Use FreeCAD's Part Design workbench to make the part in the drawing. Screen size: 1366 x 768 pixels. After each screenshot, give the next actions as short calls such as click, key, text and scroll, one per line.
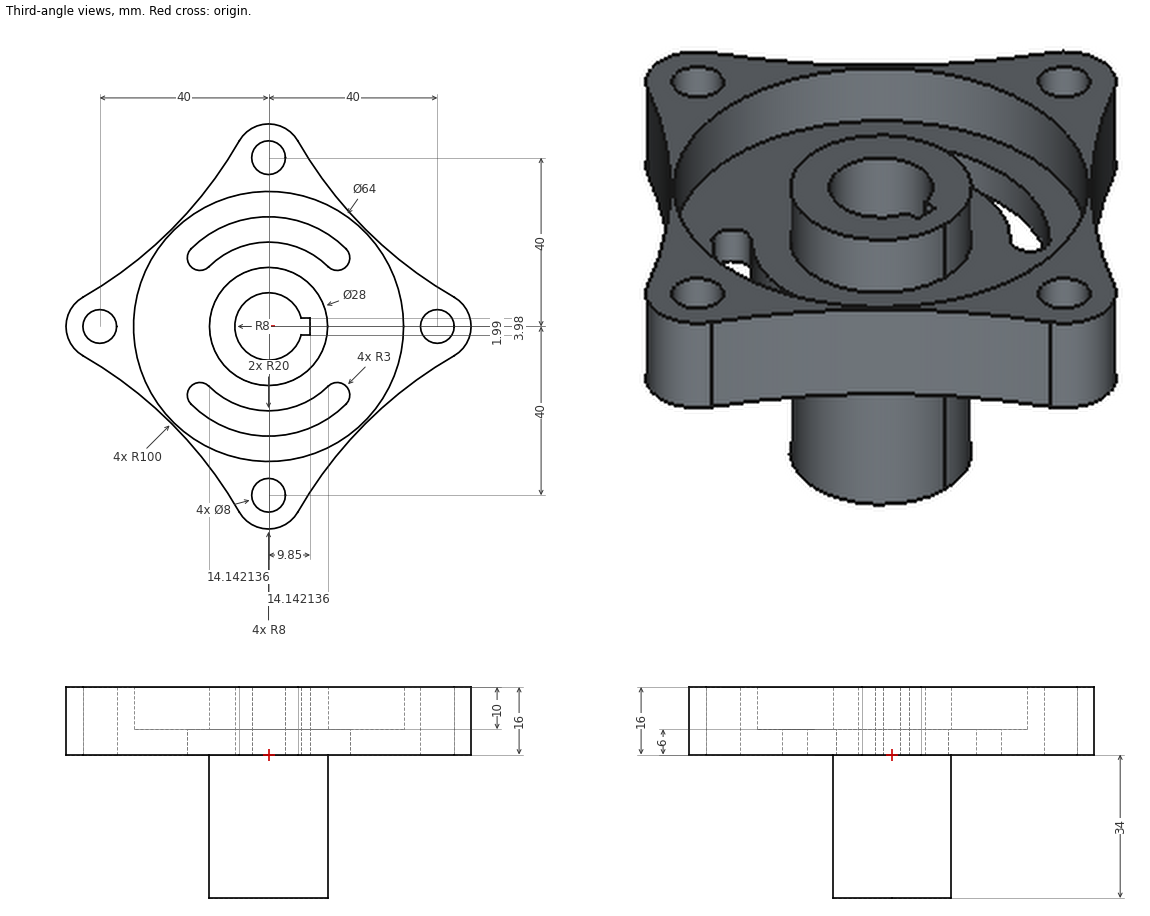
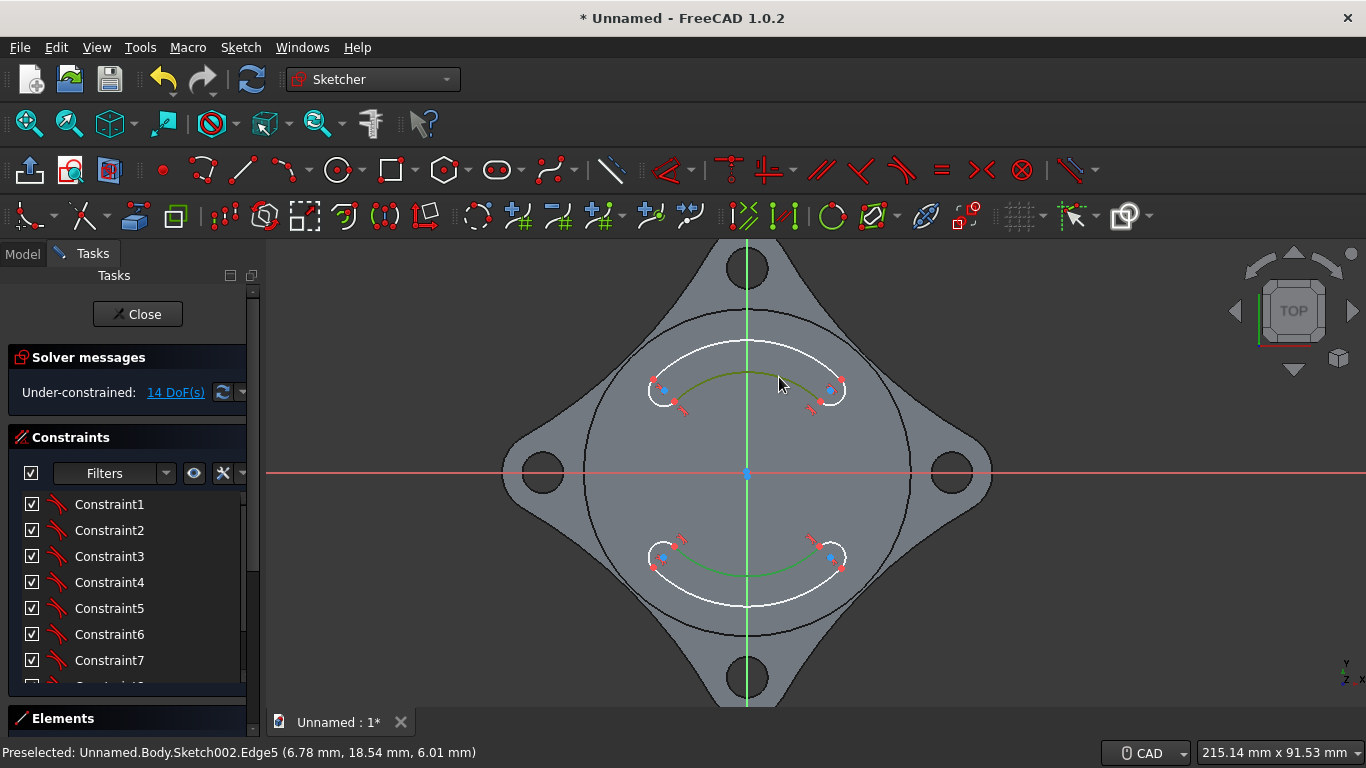
click(730, 170)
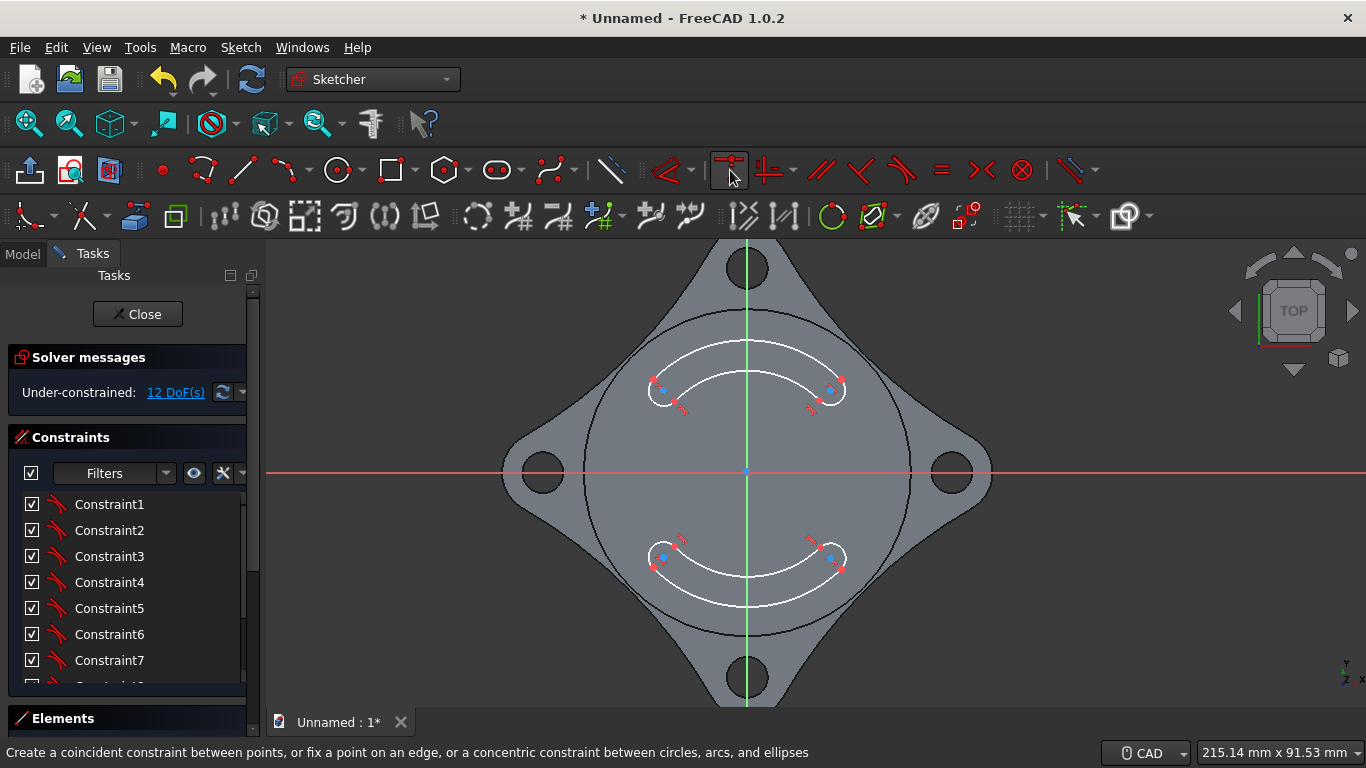
click(715, 572)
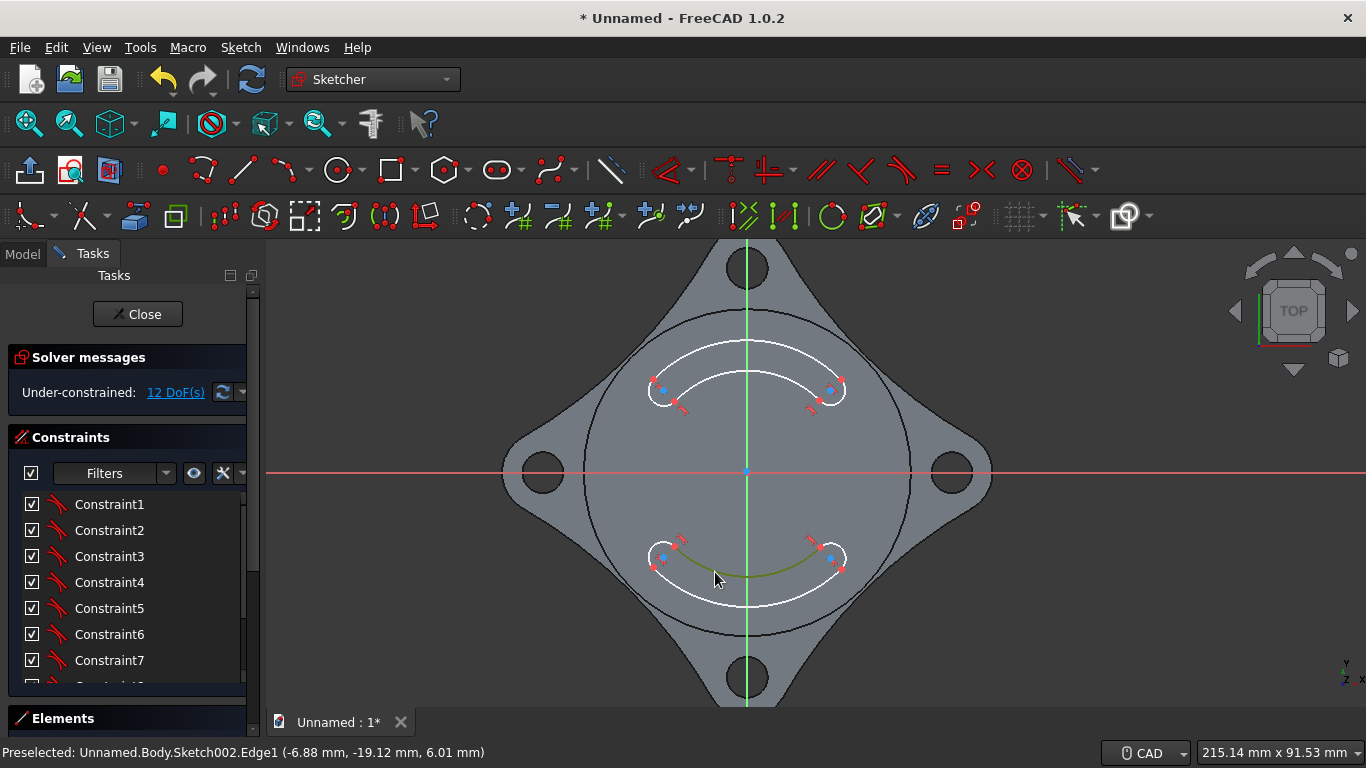
click(788, 347)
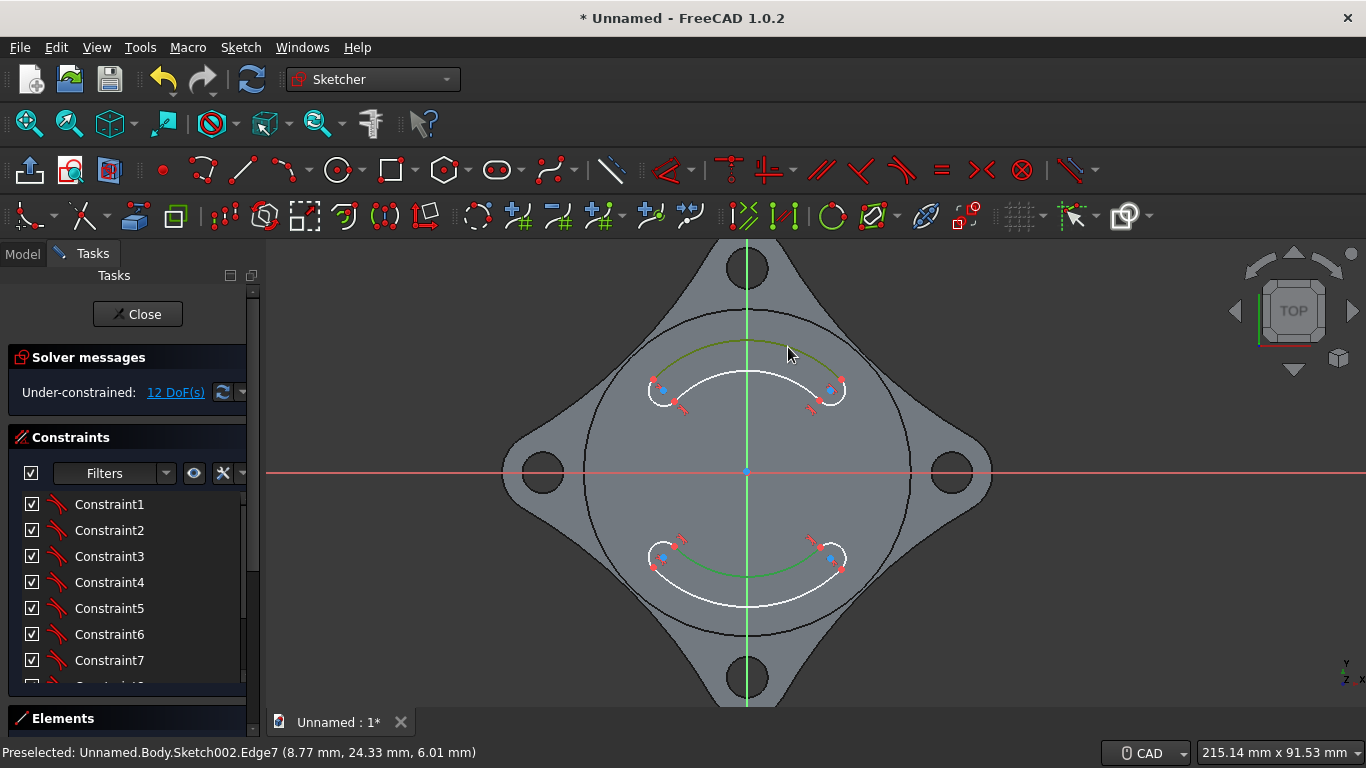
click(730, 170)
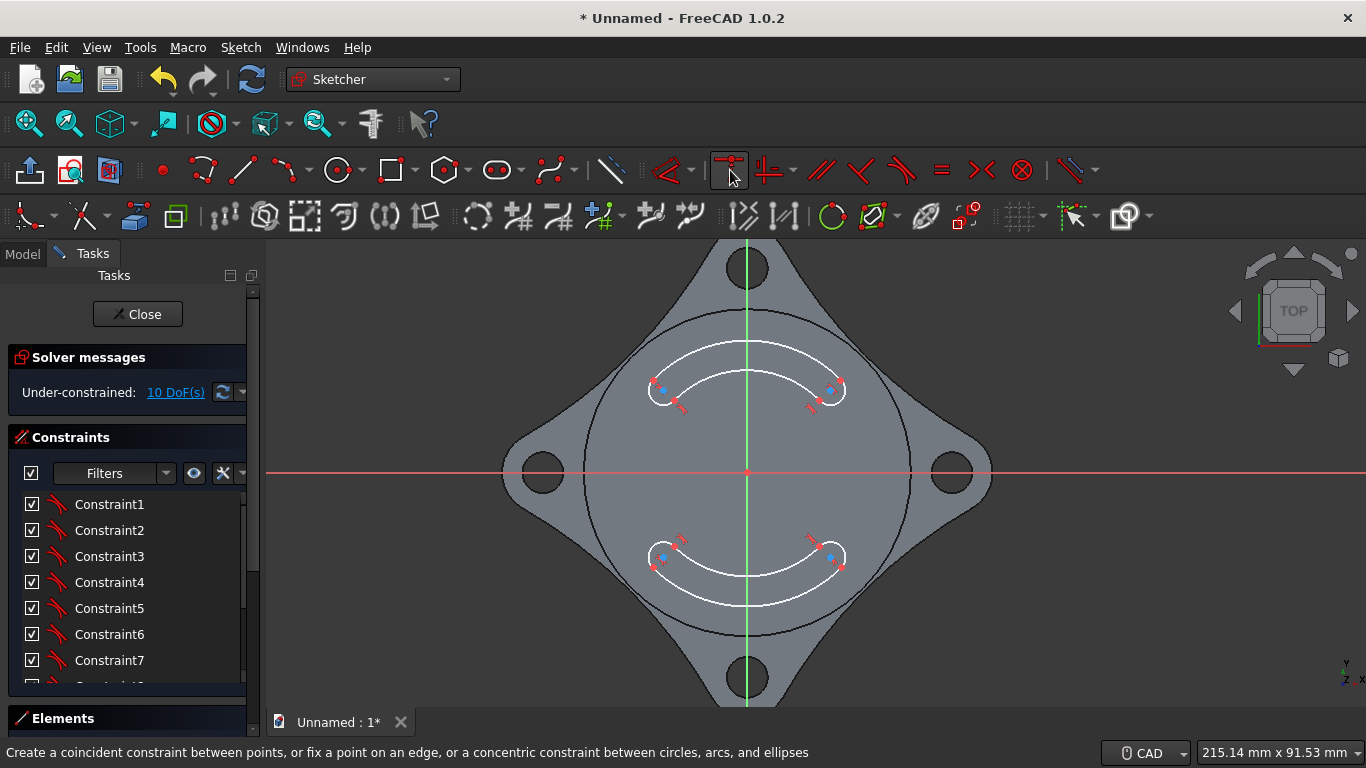
scroll(747, 473, up, 5)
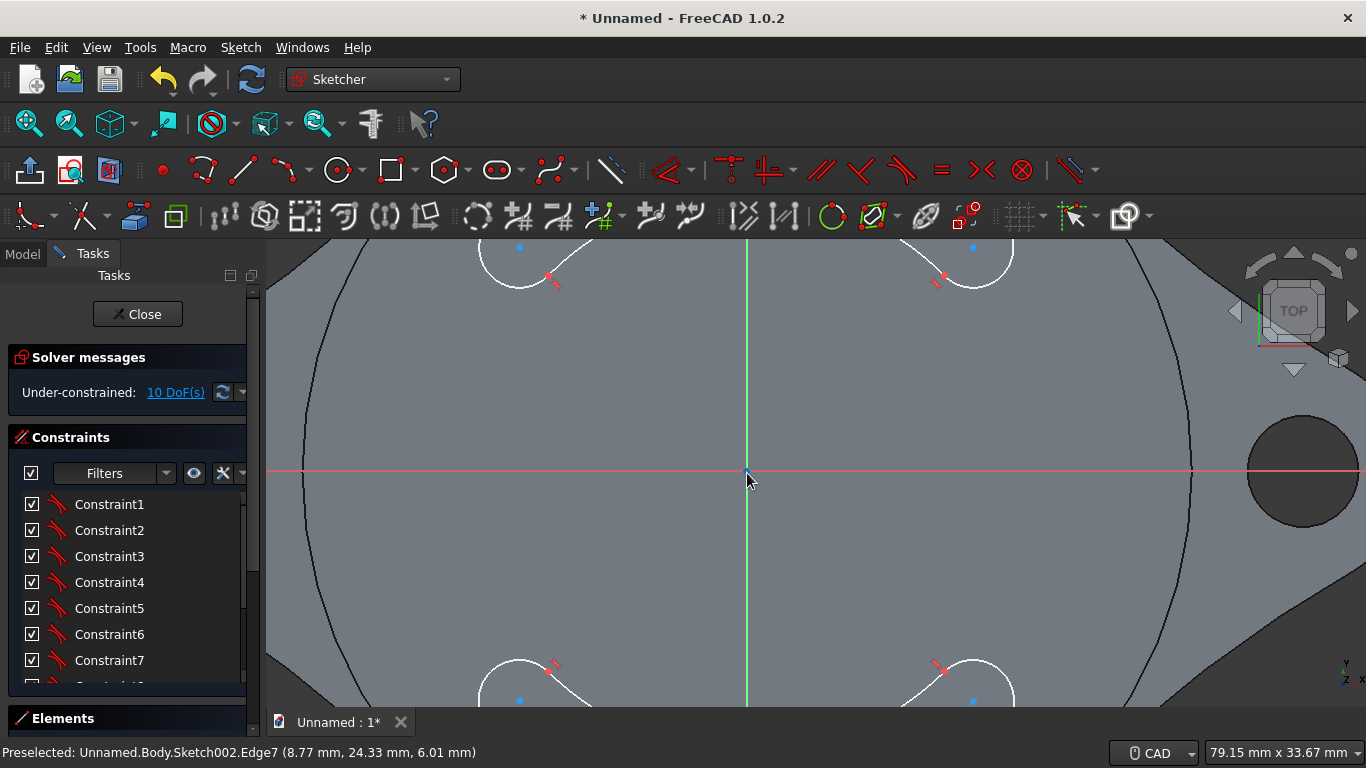
drag(736, 461, 757, 481)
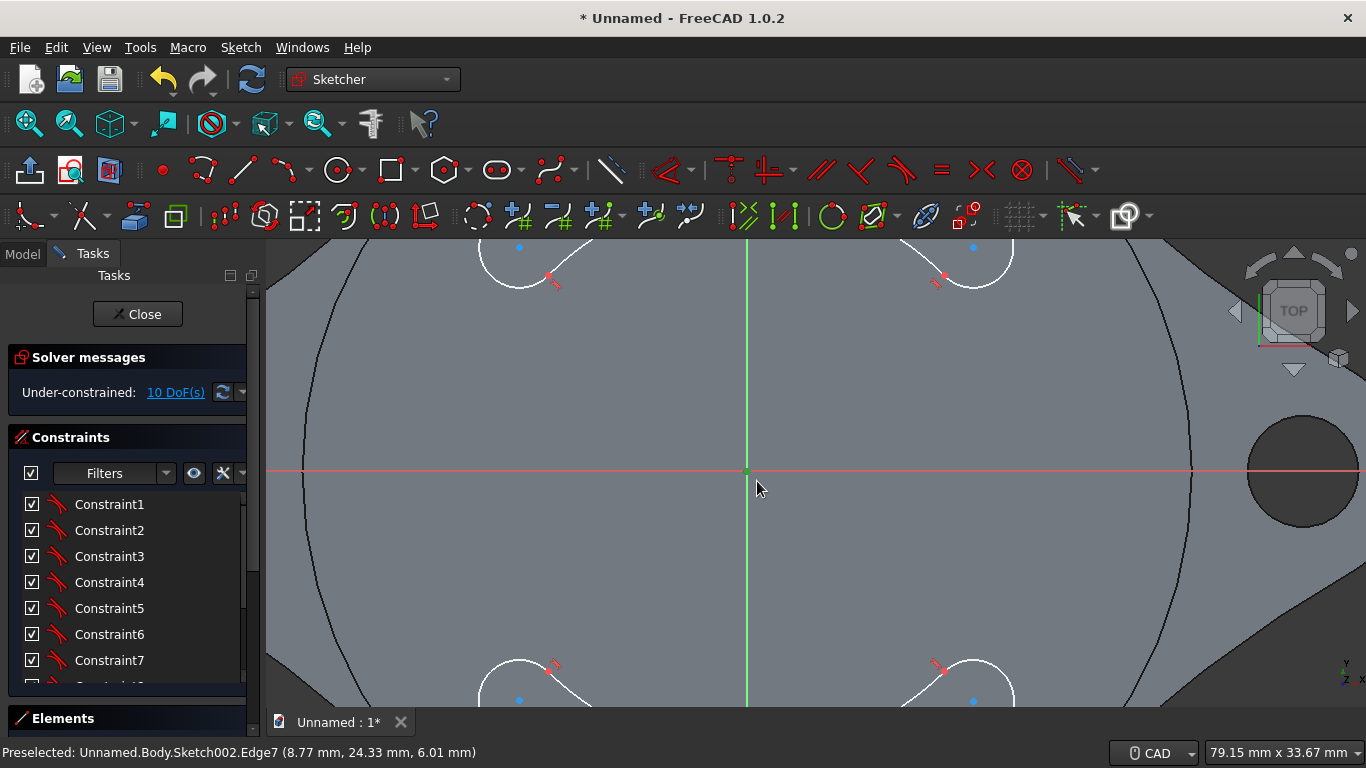
click(730, 170)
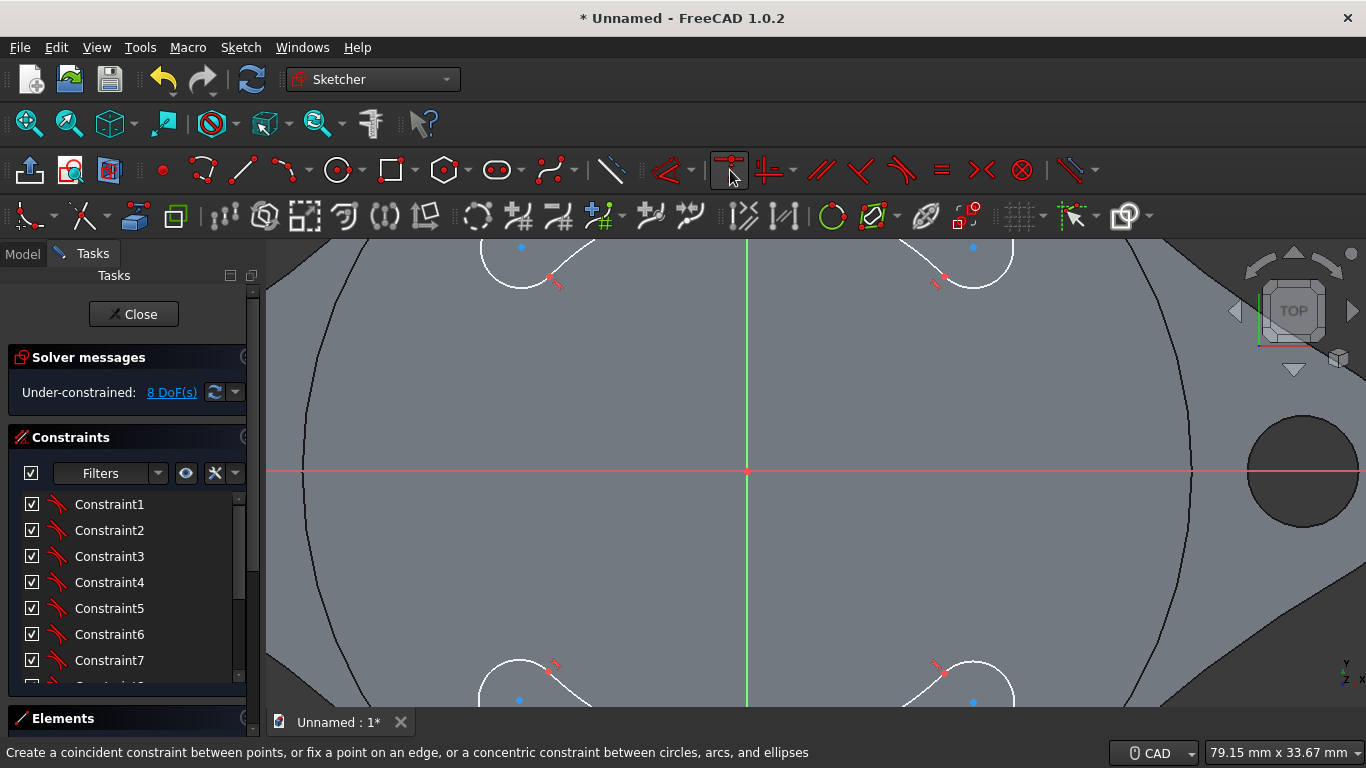
scroll(748, 474, down, 5)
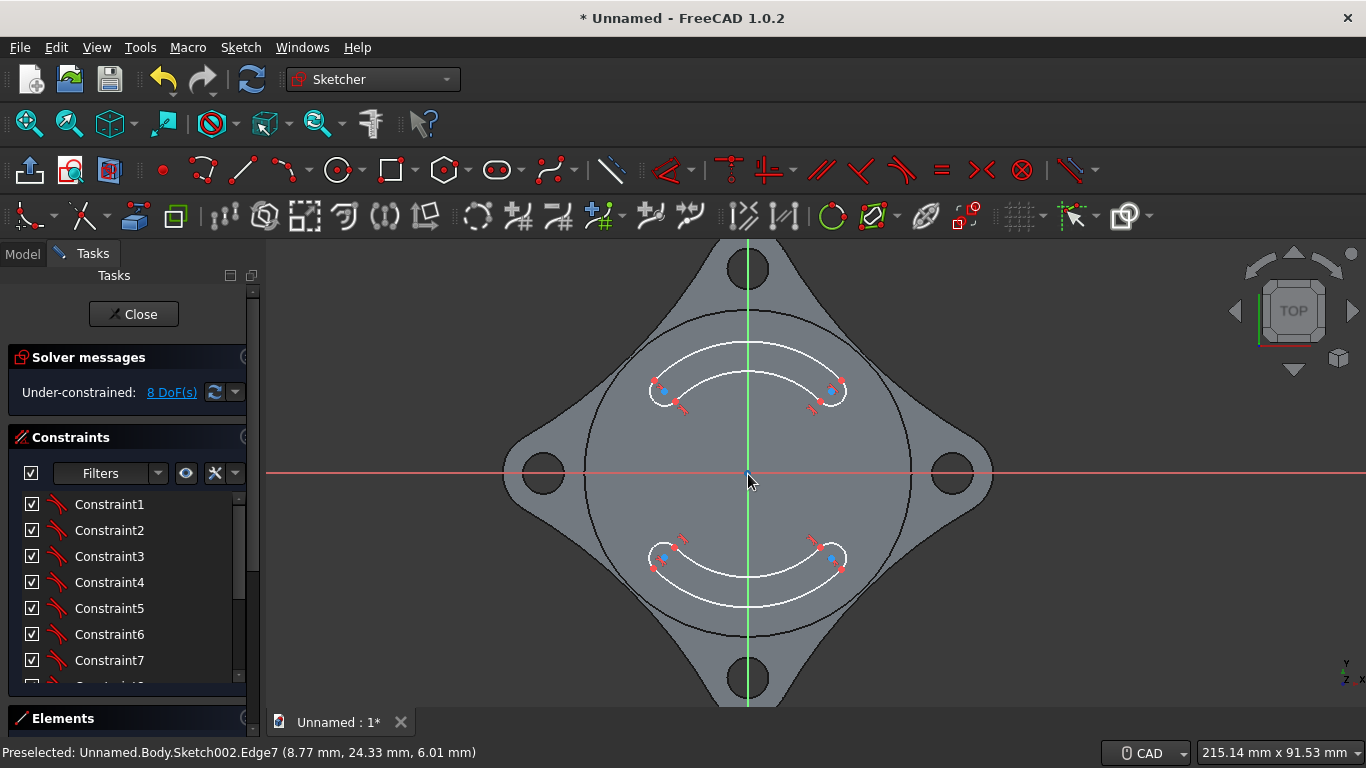
click(716, 572)